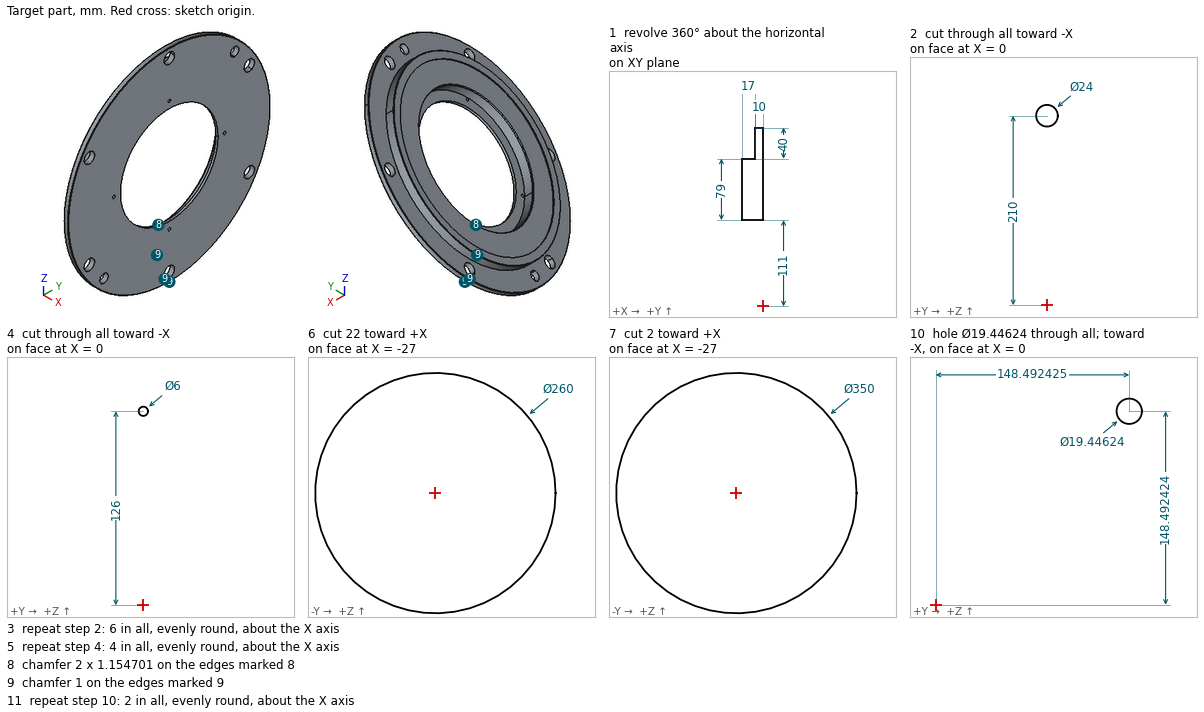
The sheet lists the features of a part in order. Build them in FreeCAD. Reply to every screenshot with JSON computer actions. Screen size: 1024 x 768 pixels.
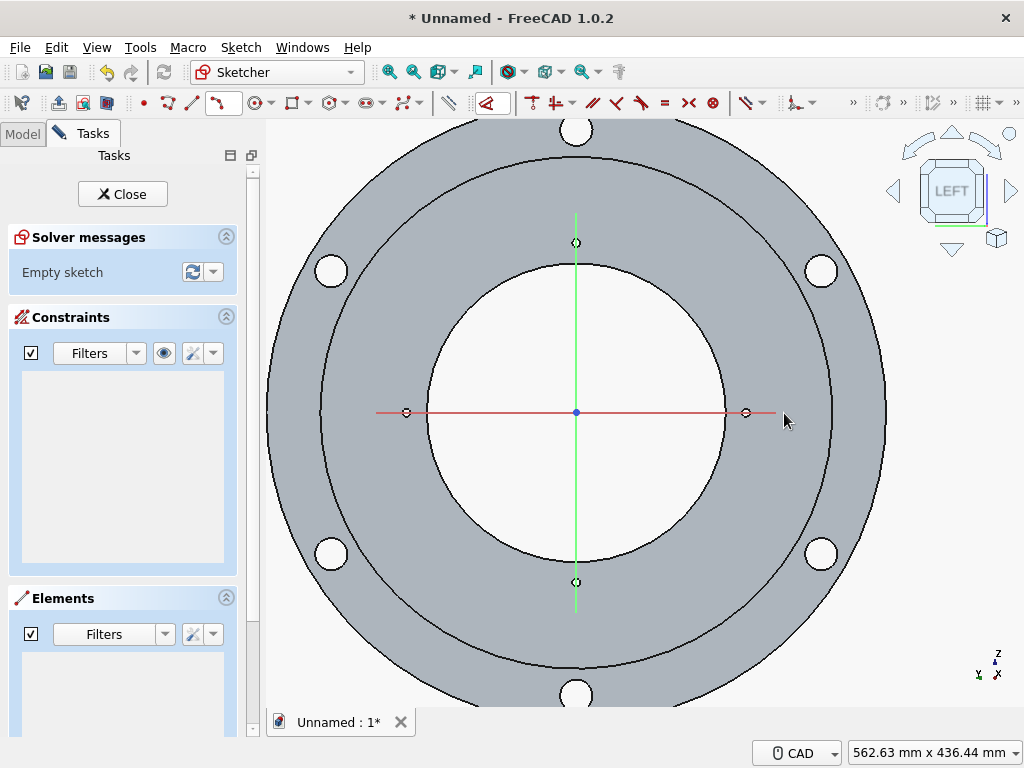
{"action": "left_click", "coordinate": [256, 104]}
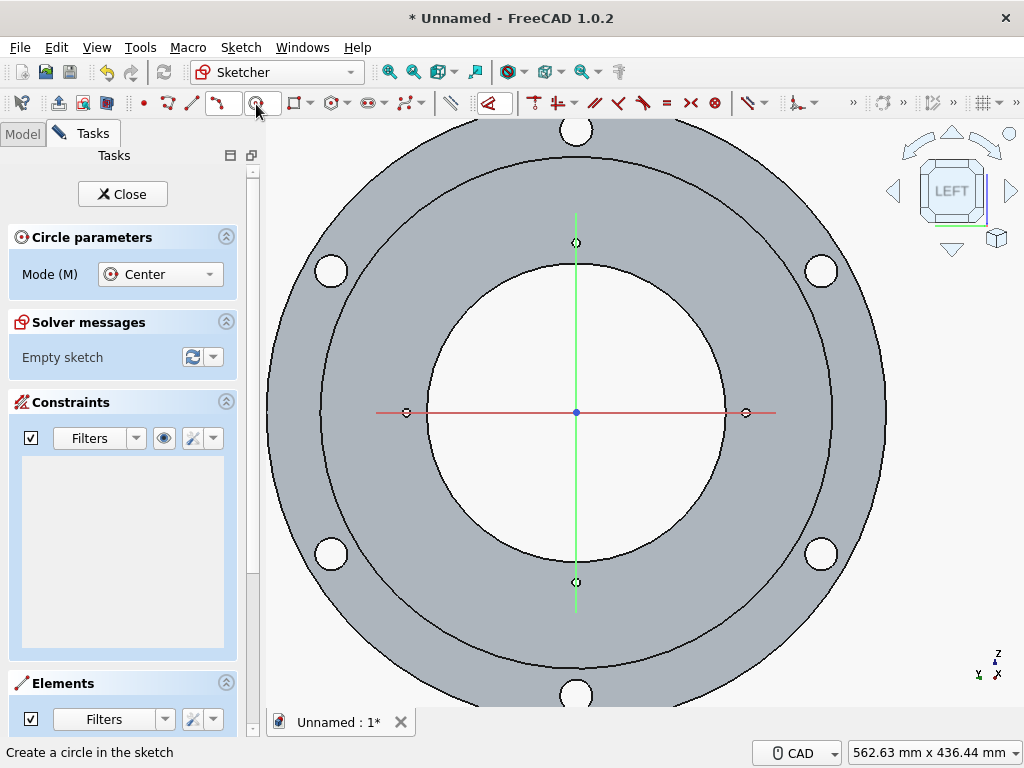
{"action": "left_click", "coordinate": [576, 413]}
{"action": "mouse_move", "coordinate": [700, 289]}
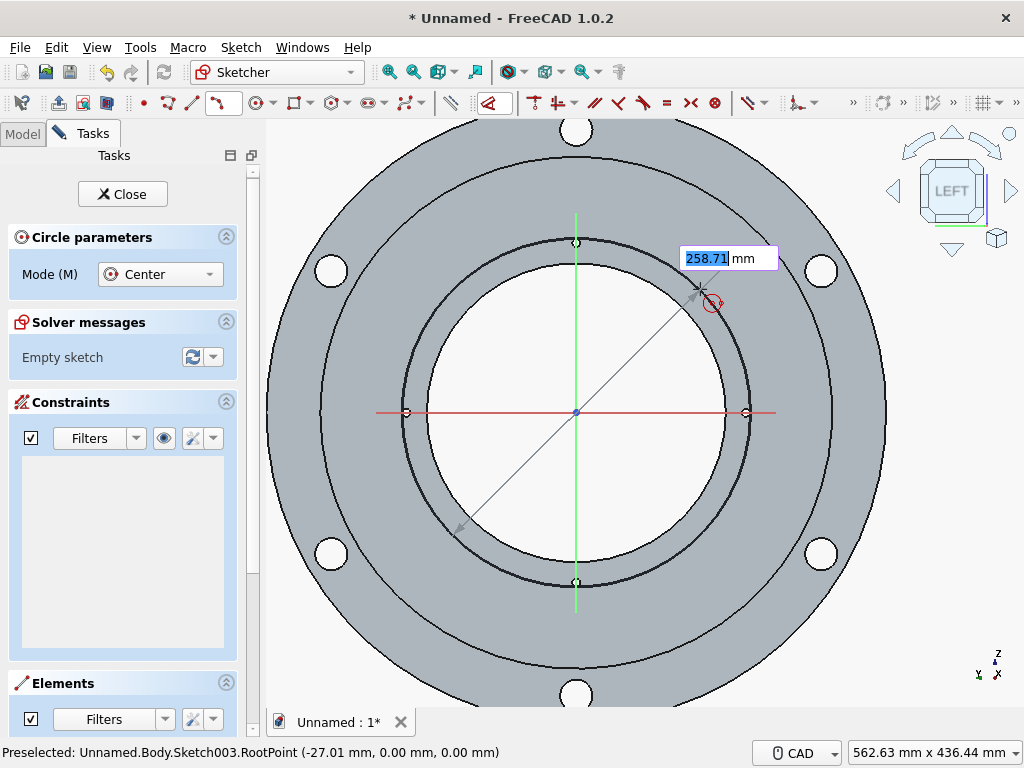
{"action": "type", "text": "260"}
{"action": "key", "text": "Return"}
{"action": "key", "text": "Escape"}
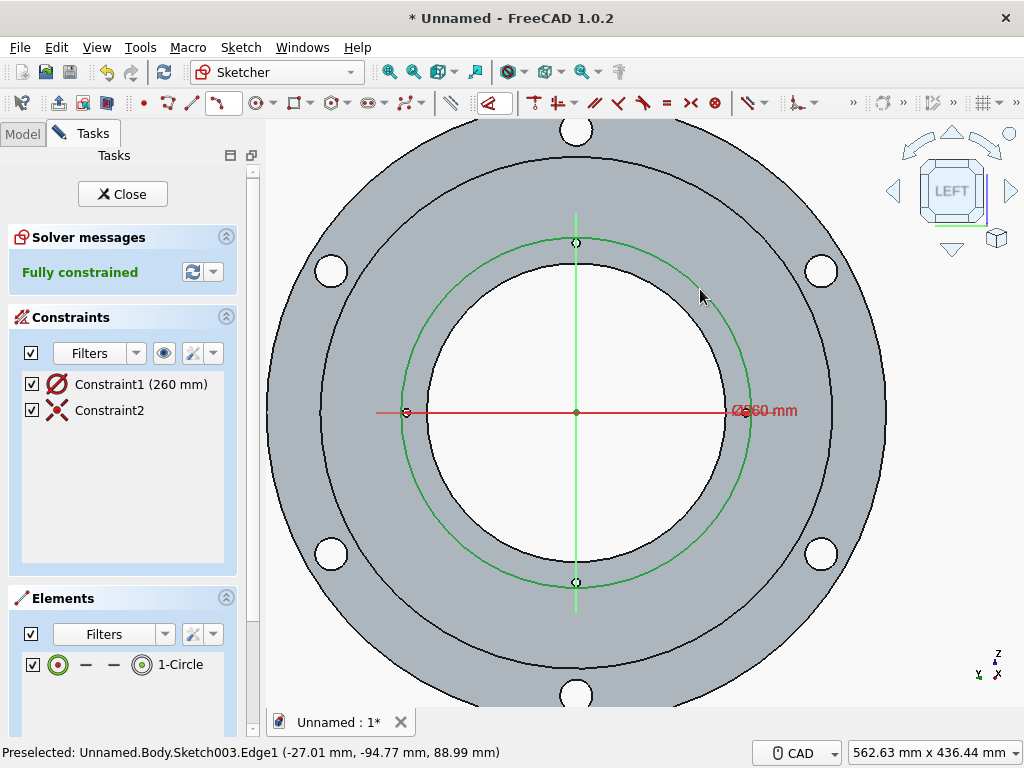
{"action": "left_click", "coordinate": [123, 194]}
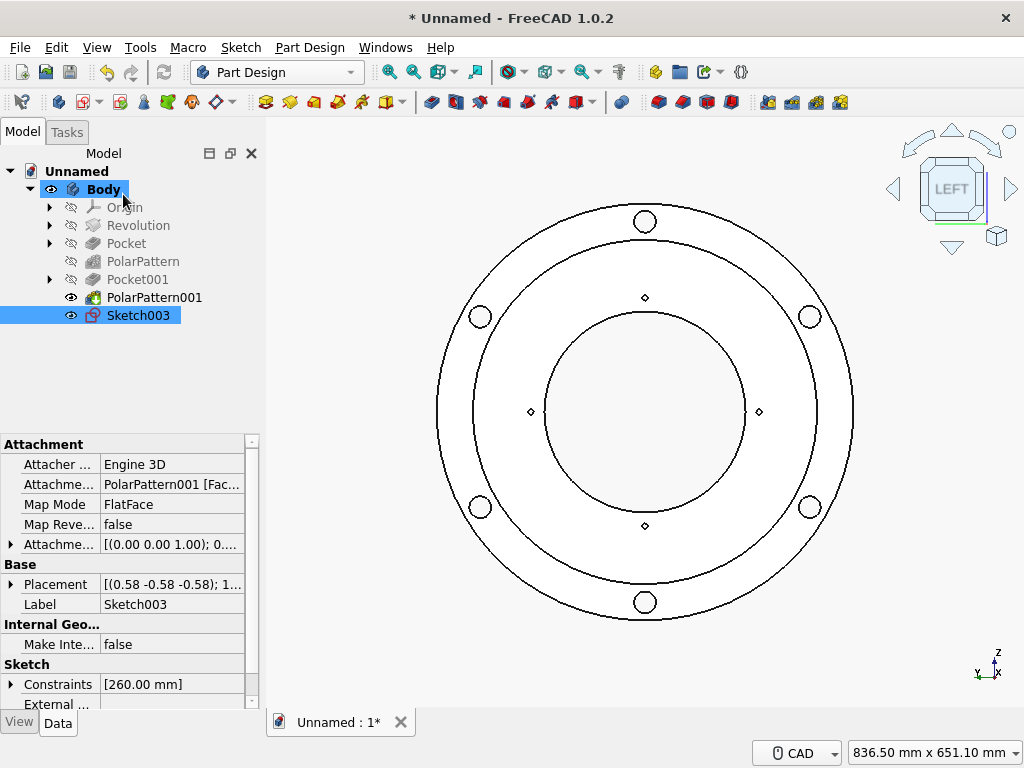
{"action": "left_click", "coordinate": [432, 102]}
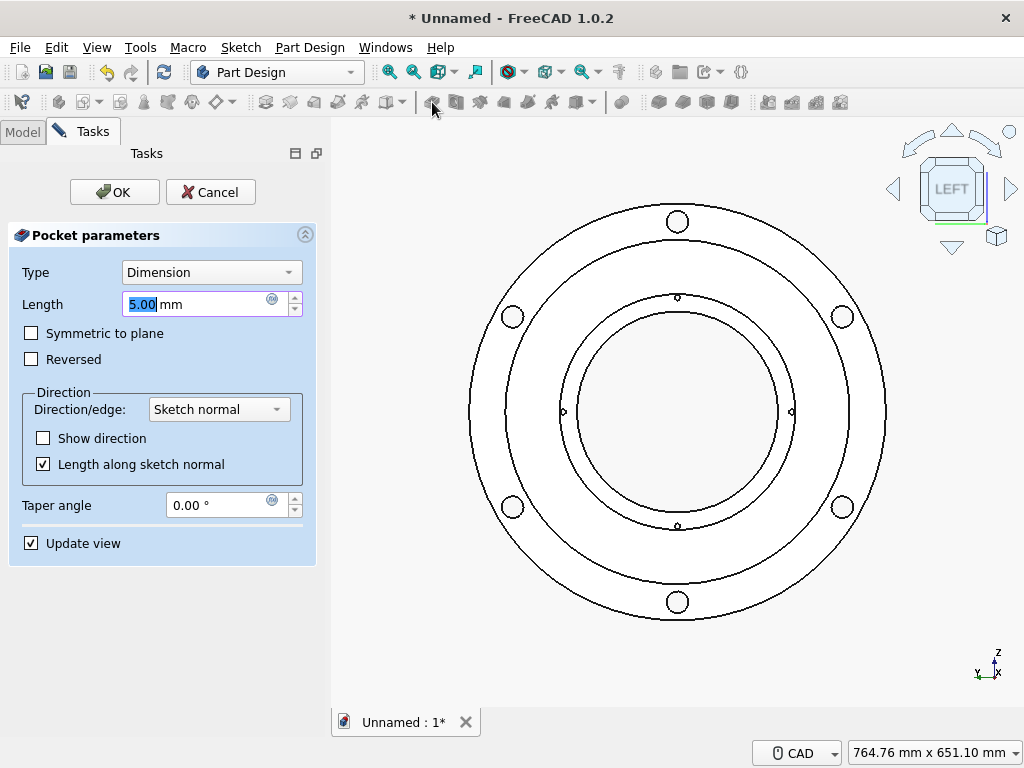
{"action": "type", "text": "22"}
{"action": "key", "text": "Tab"}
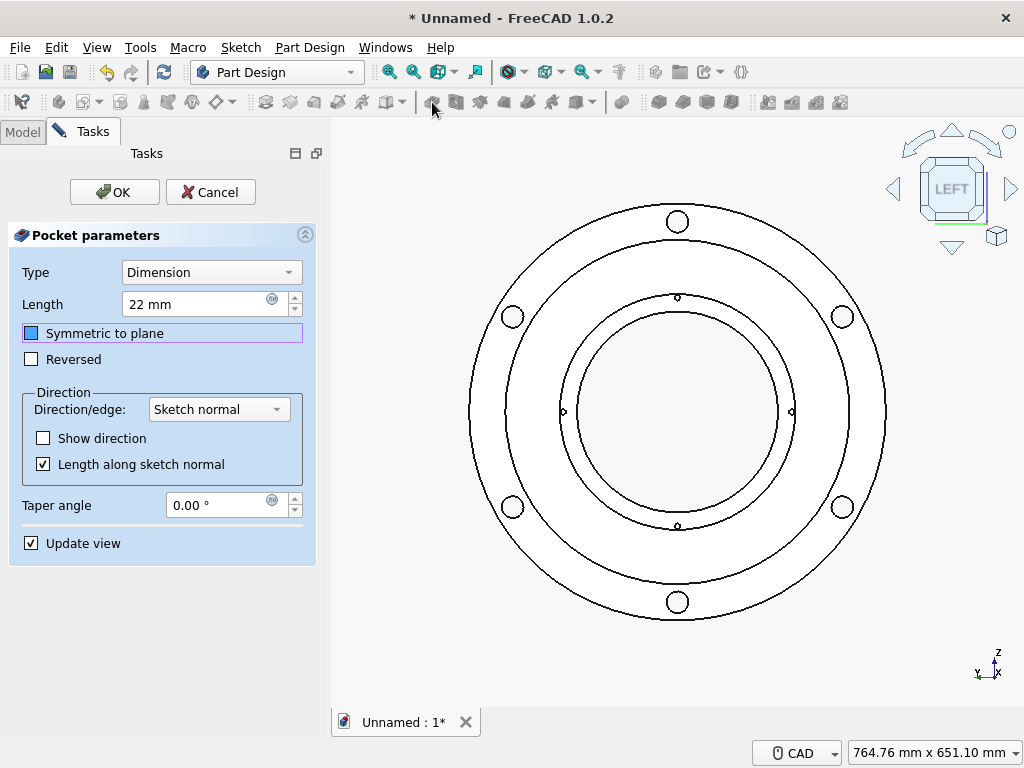
{"action": "left_click", "coordinate": [115, 192]}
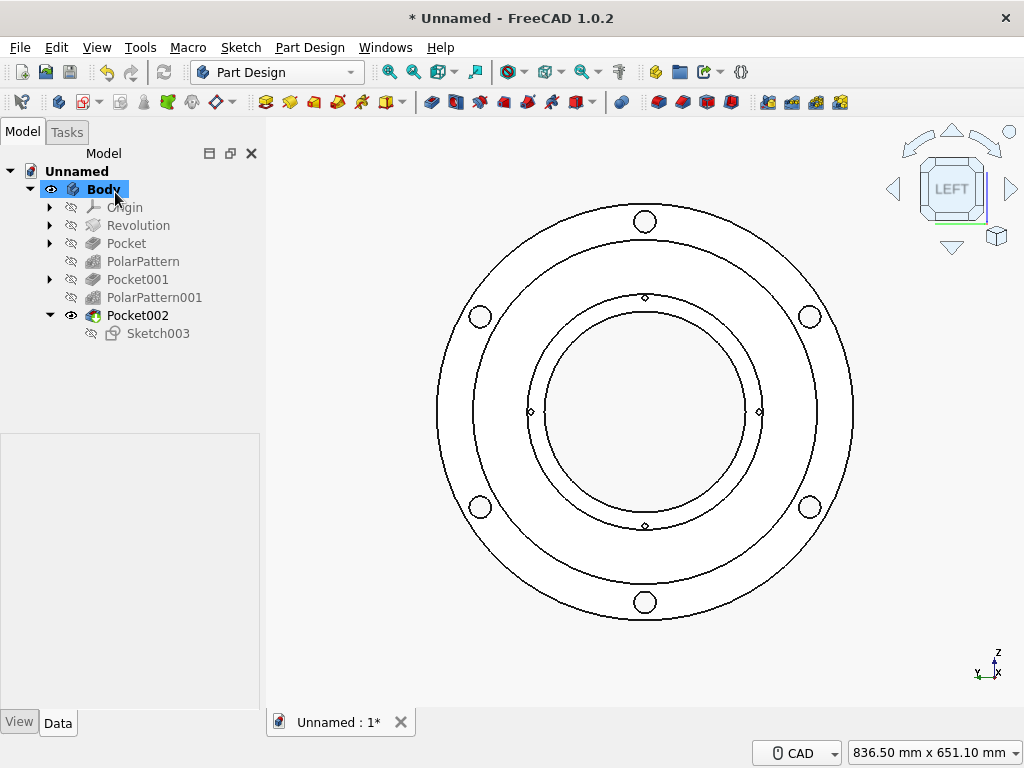
{"action": "left_click", "coordinate": [497, 411]}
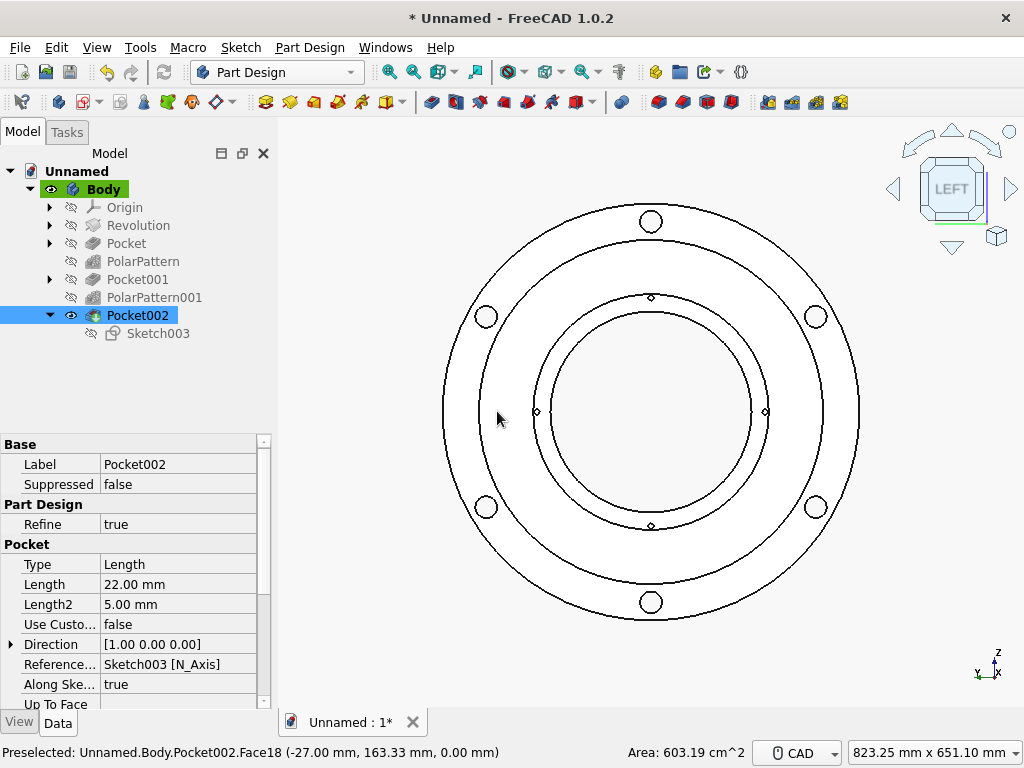
{"action": "left_click", "coordinate": [84, 102]}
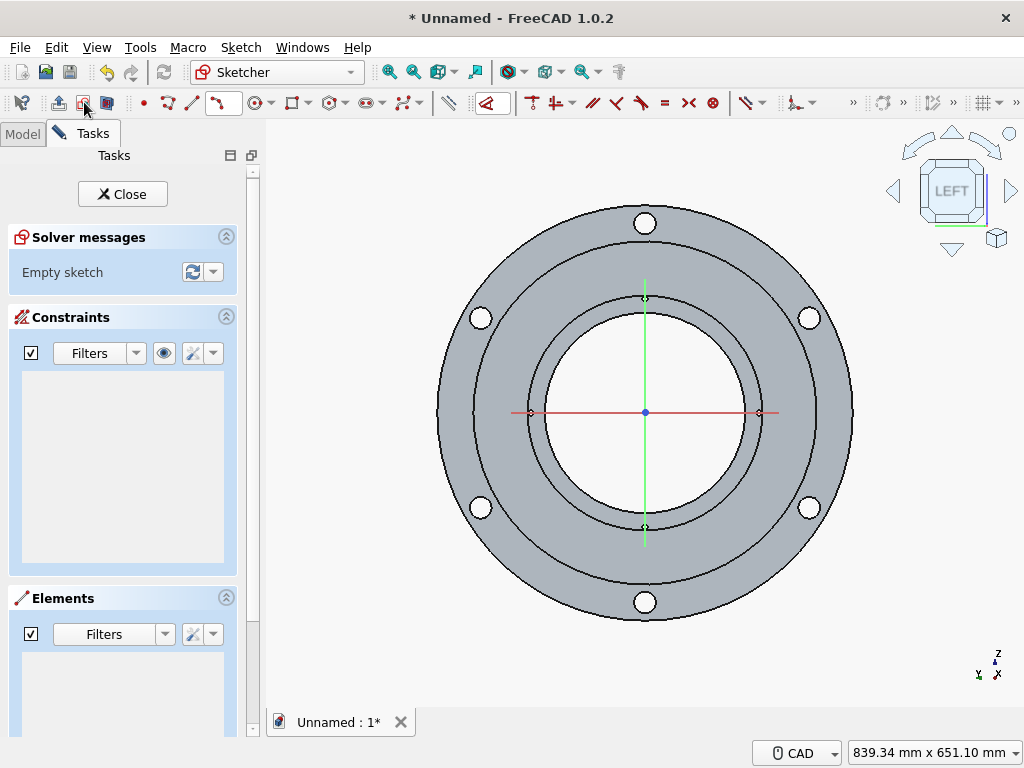
{"action": "left_click", "coordinate": [256, 104]}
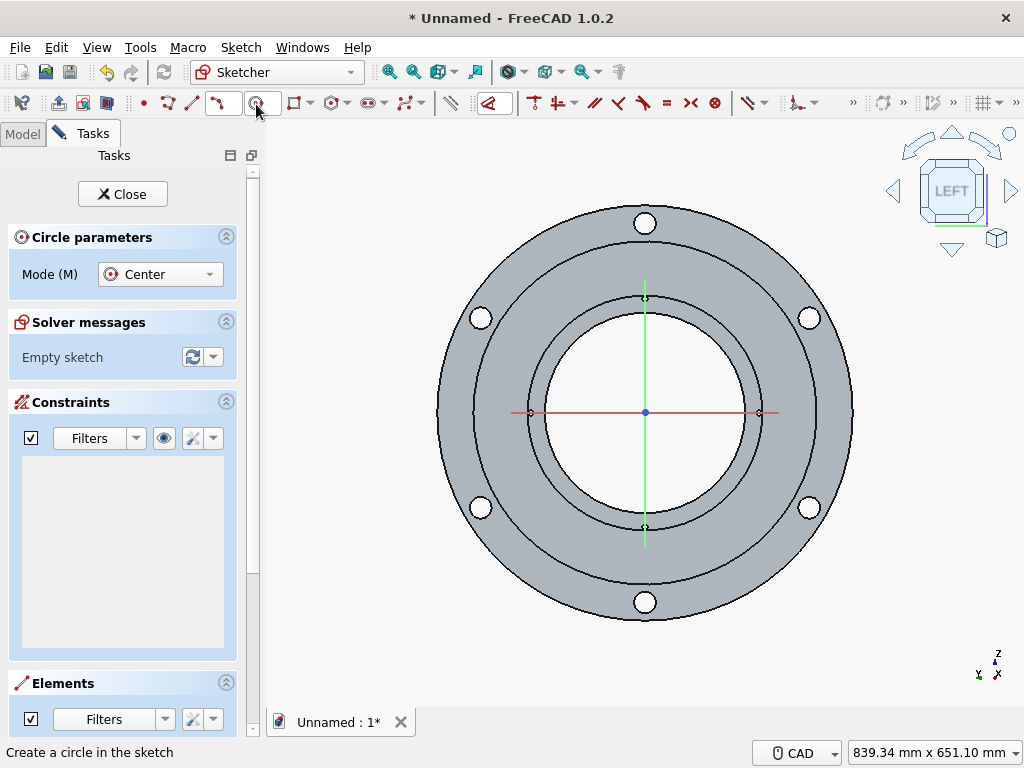
{"action": "left_click", "coordinate": [645, 413]}
{"action": "mouse_move", "coordinate": [757, 301]}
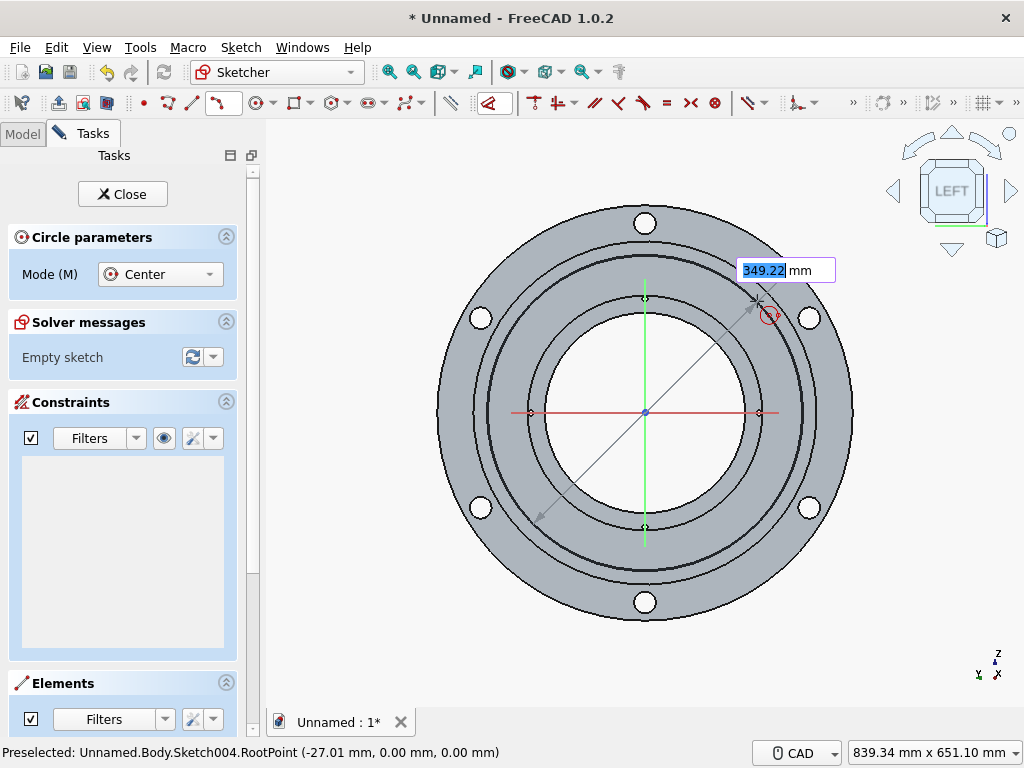
{"action": "type", "text": "350"}
{"action": "key", "text": "Return"}
{"action": "key", "text": "Escape"}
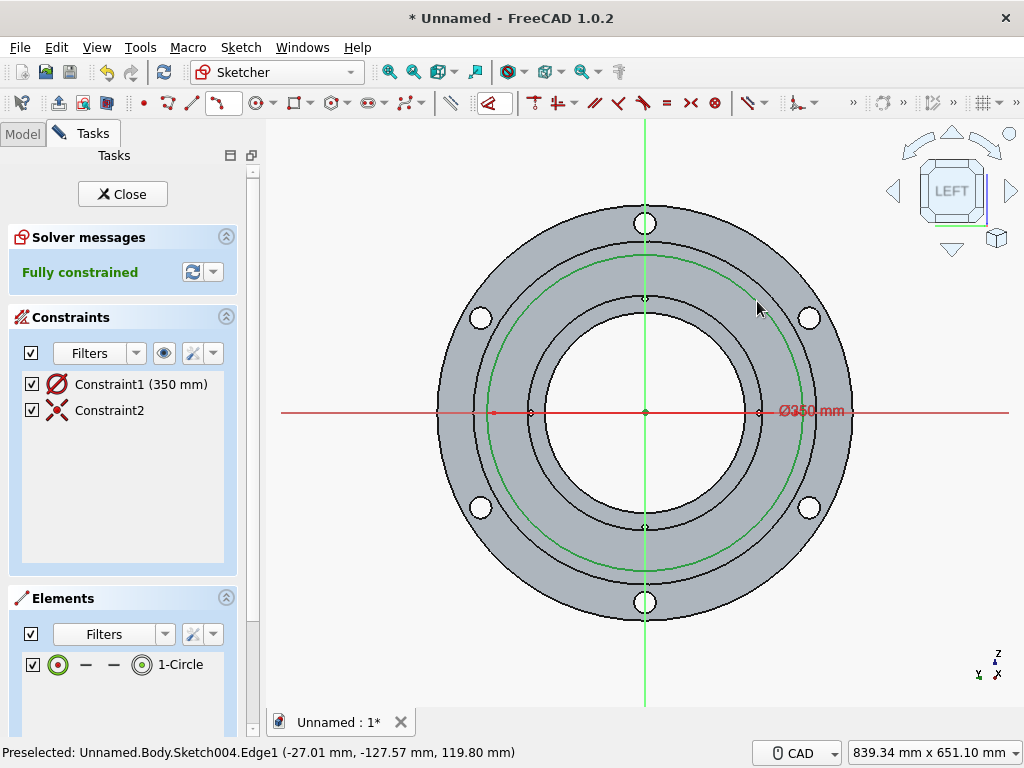
{"action": "left_click", "coordinate": [123, 194]}